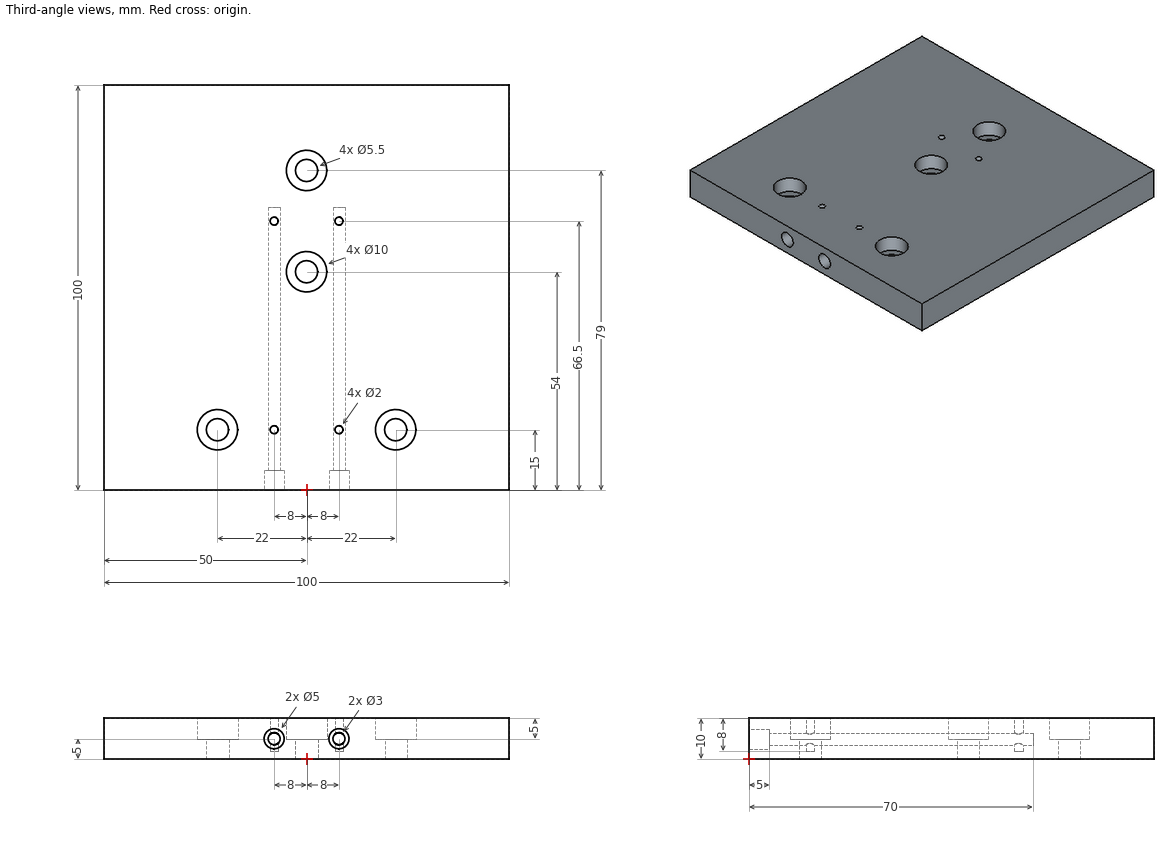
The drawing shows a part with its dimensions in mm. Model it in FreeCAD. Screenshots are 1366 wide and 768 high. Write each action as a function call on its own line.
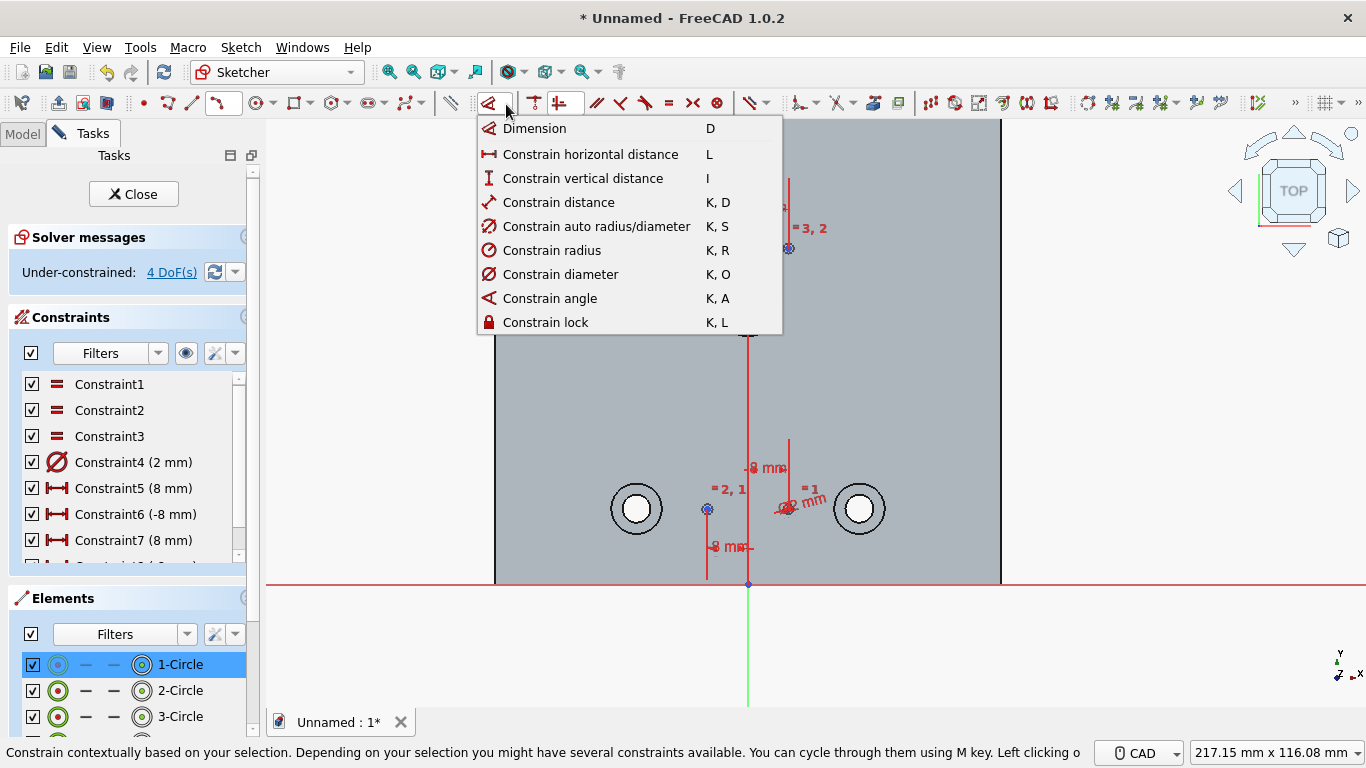
click(630, 178)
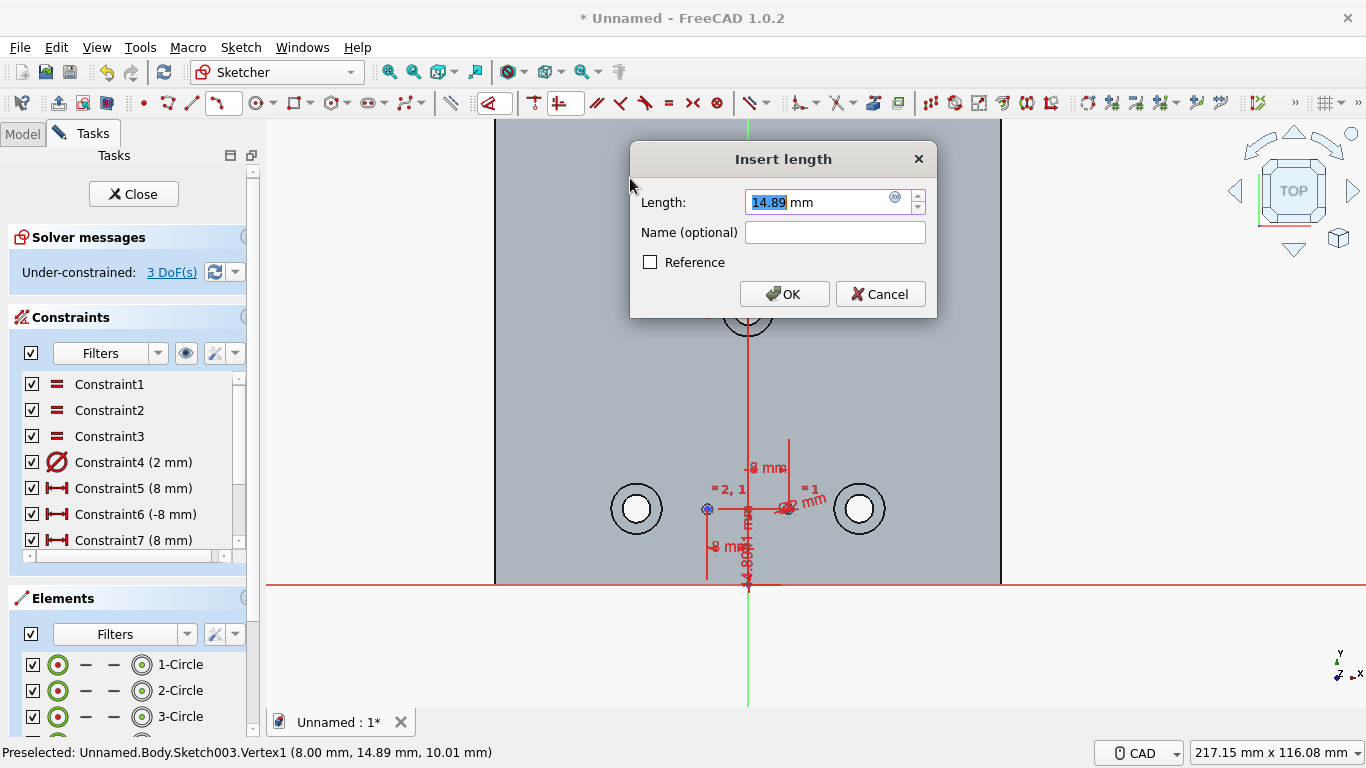
text(15)
key(Return)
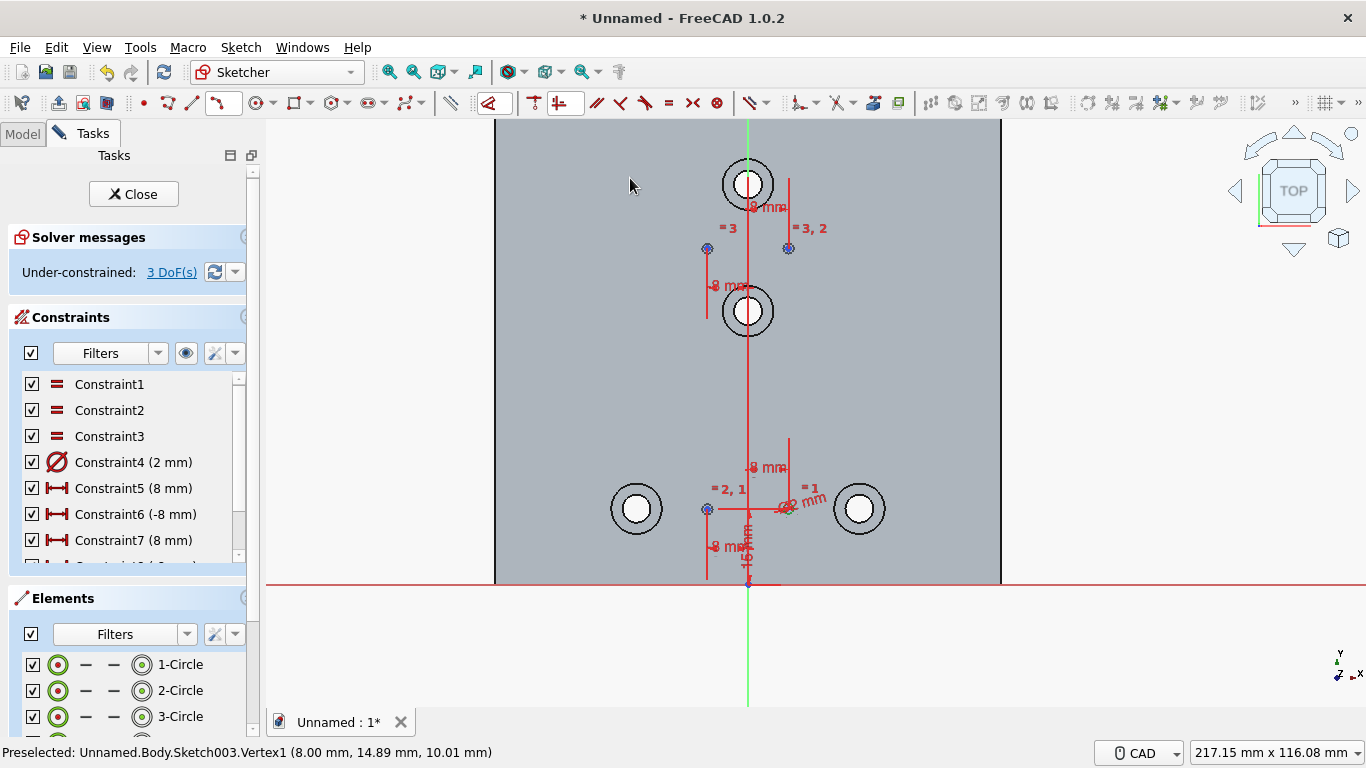
click(707, 509)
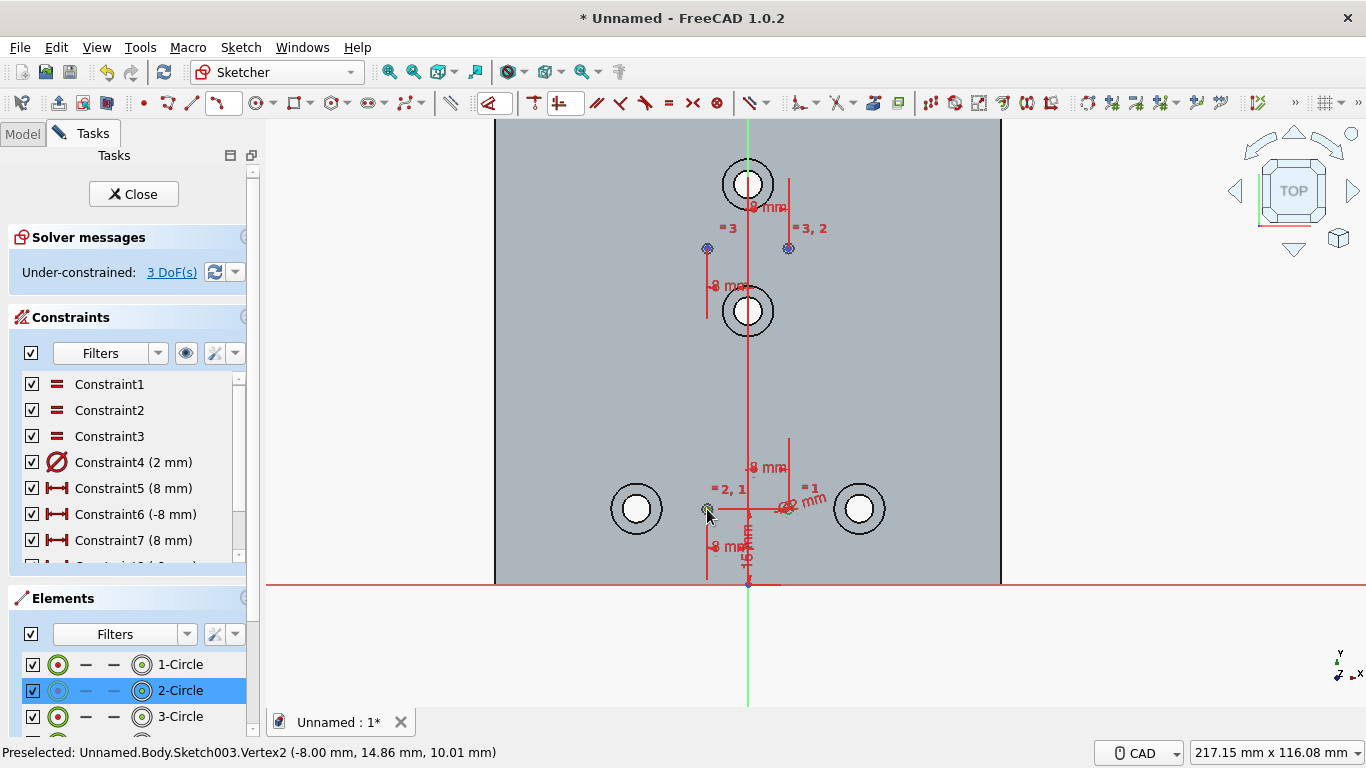
click(506, 104)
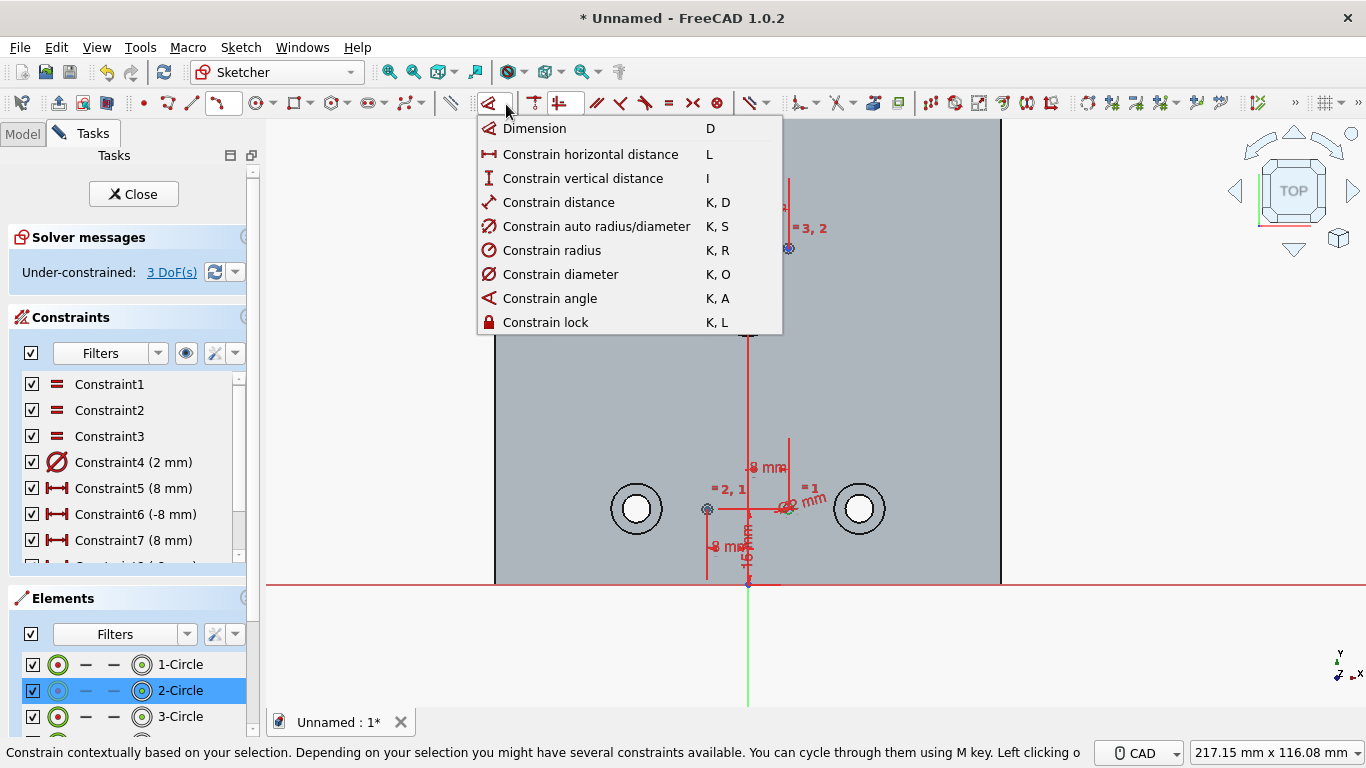
click(630, 178)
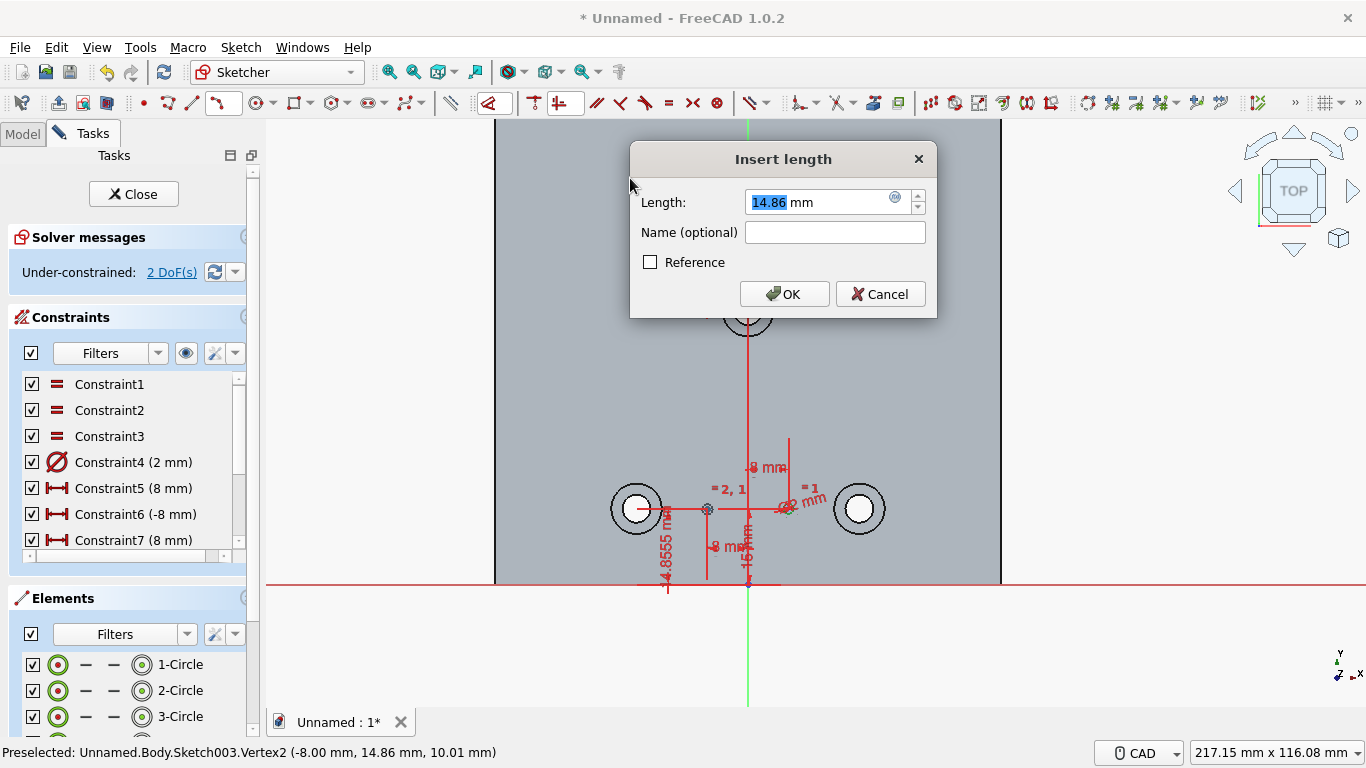
text(15)
key(Return)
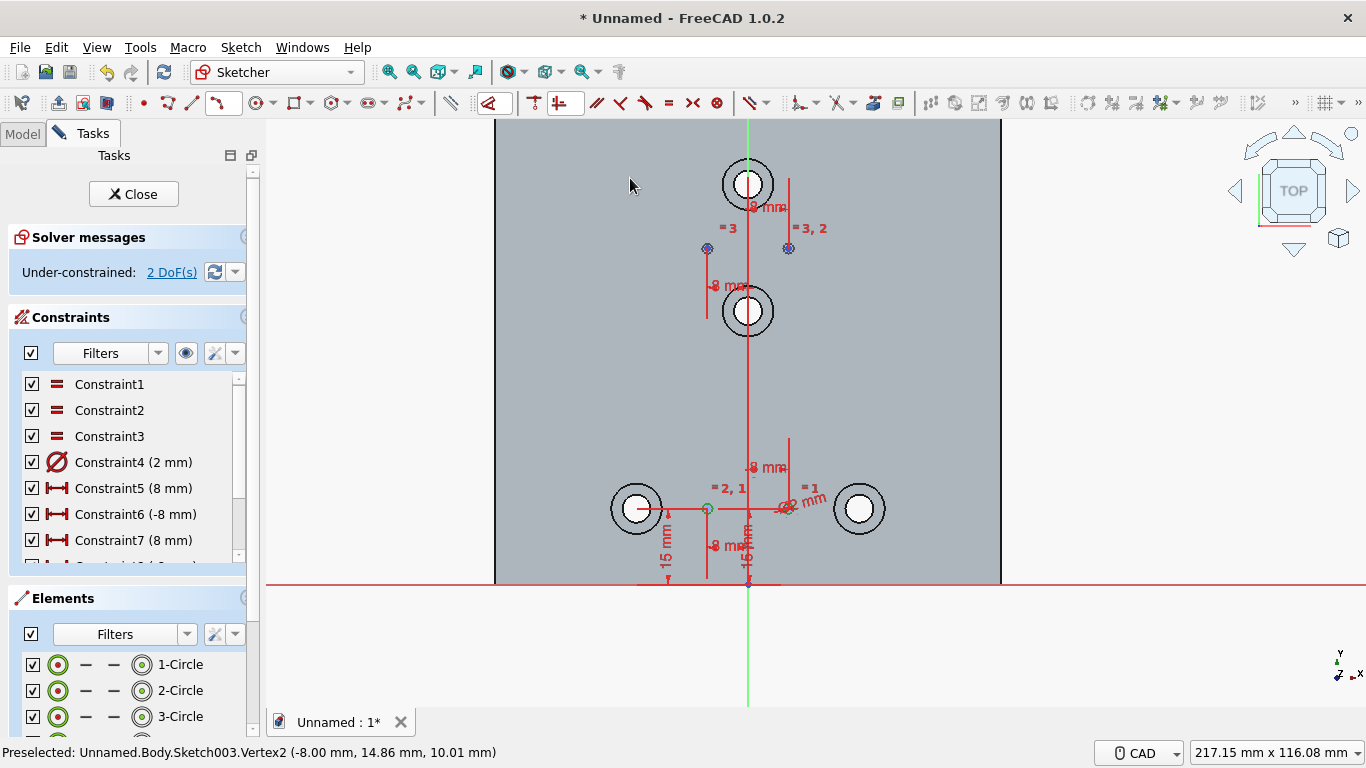
click(789, 248)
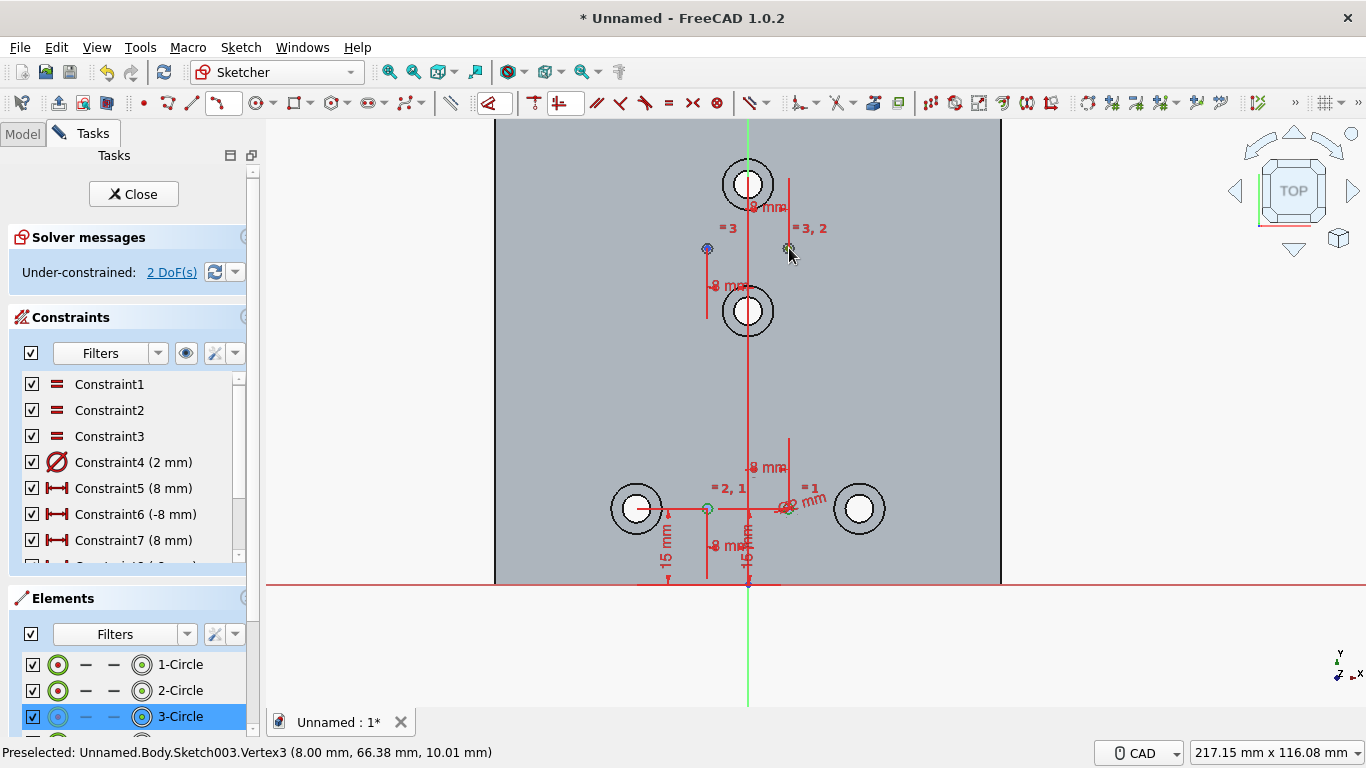
key(i)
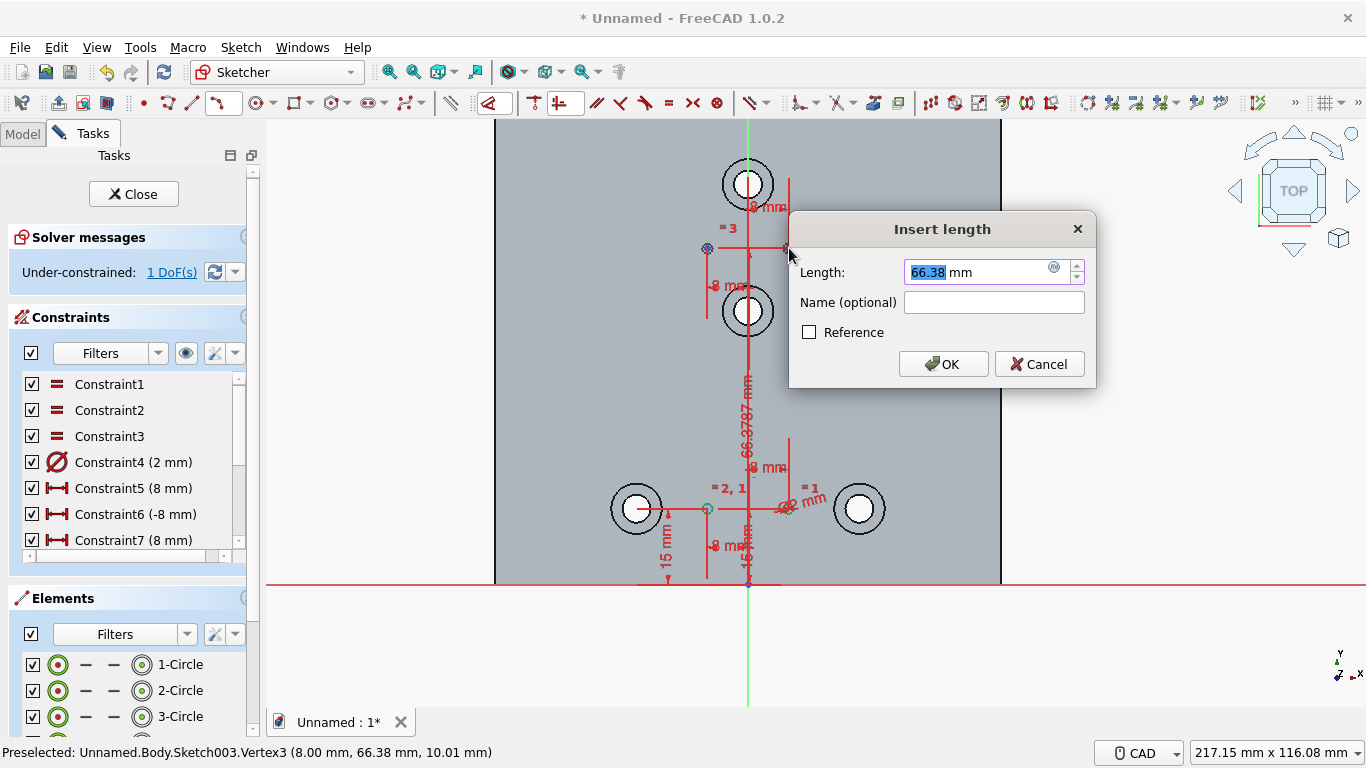
text(66.5)
key(Return)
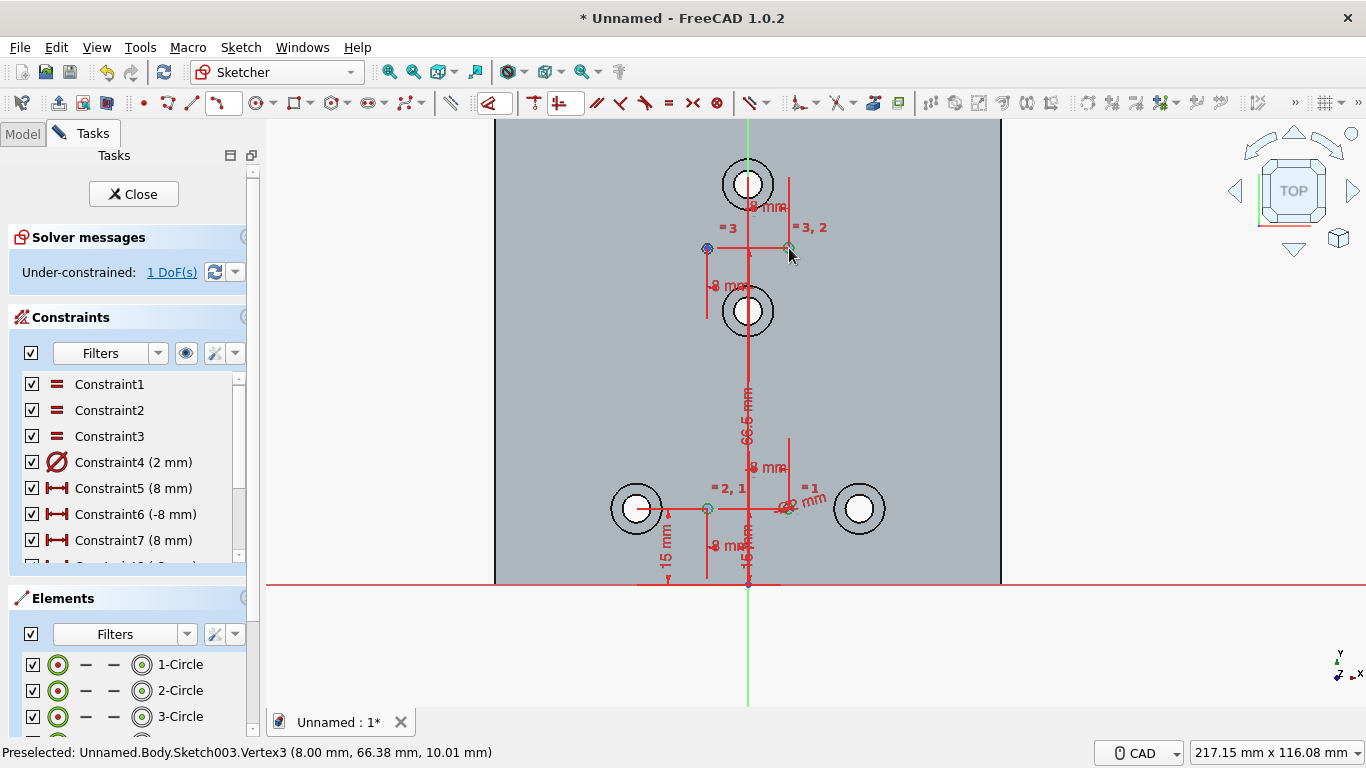
click(707, 249)